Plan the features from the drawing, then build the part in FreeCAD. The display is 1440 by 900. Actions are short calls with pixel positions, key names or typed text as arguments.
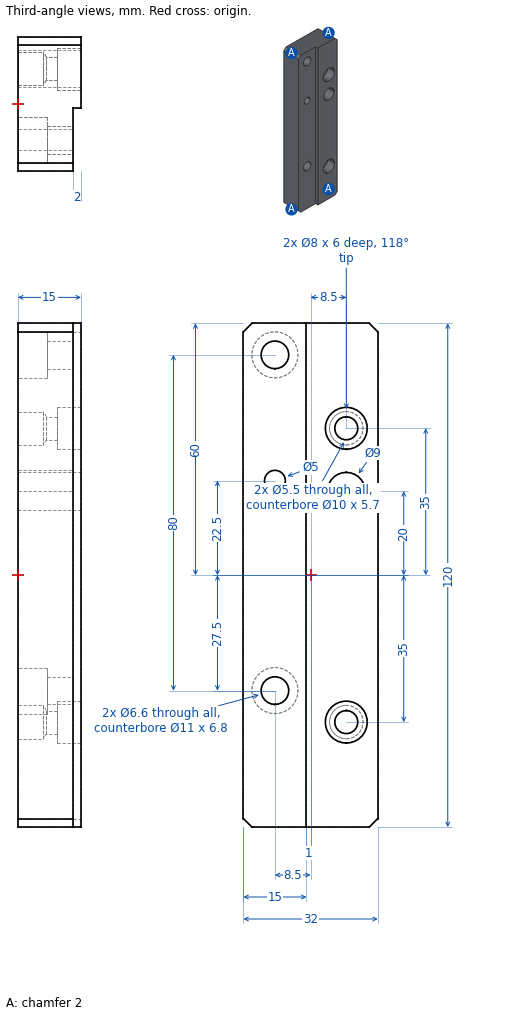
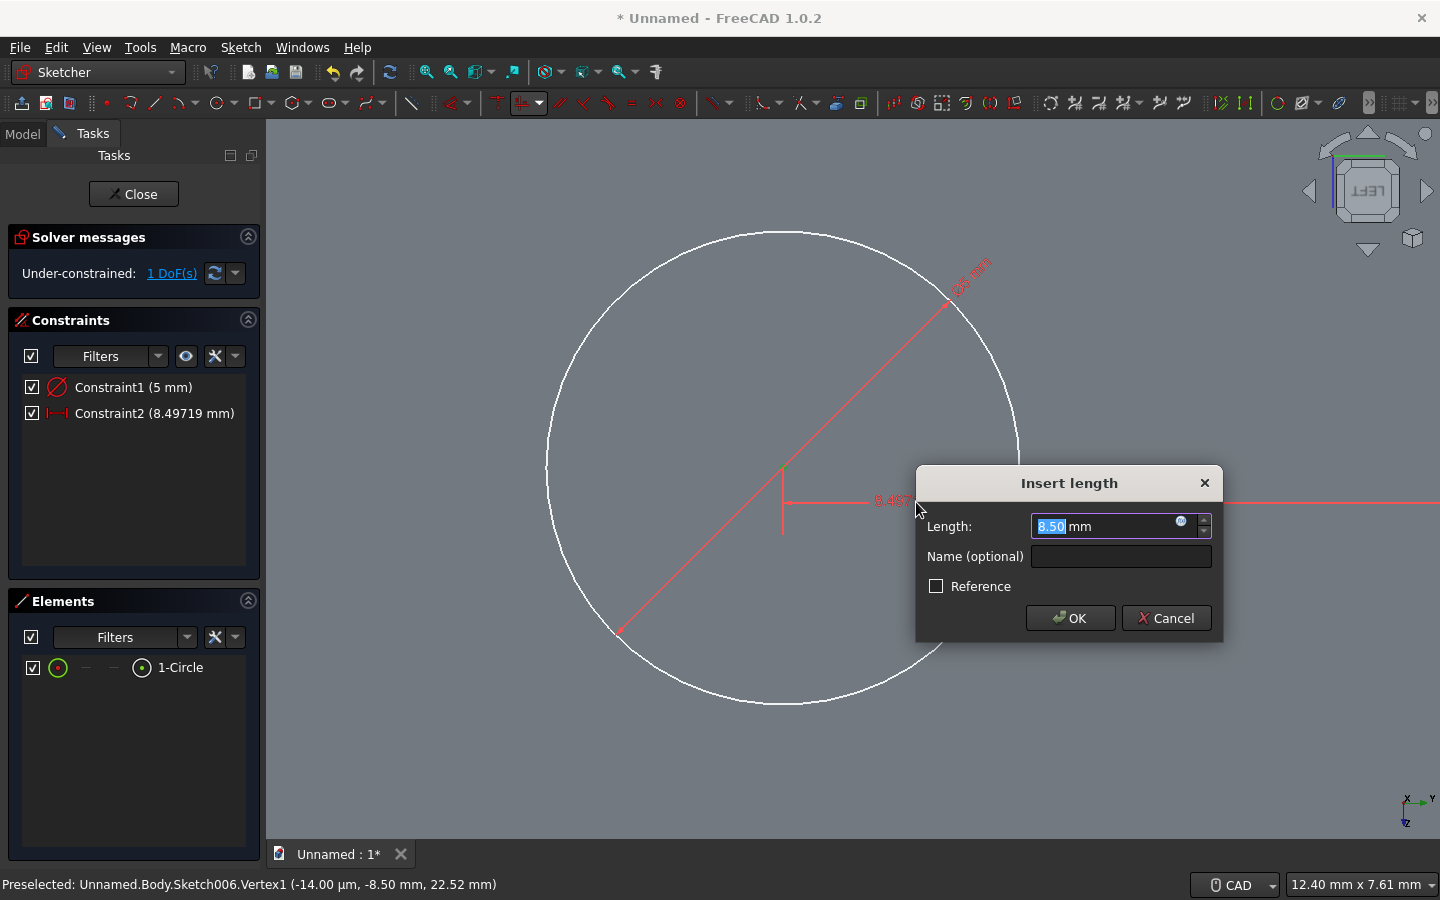
text(8.5)
key(Return)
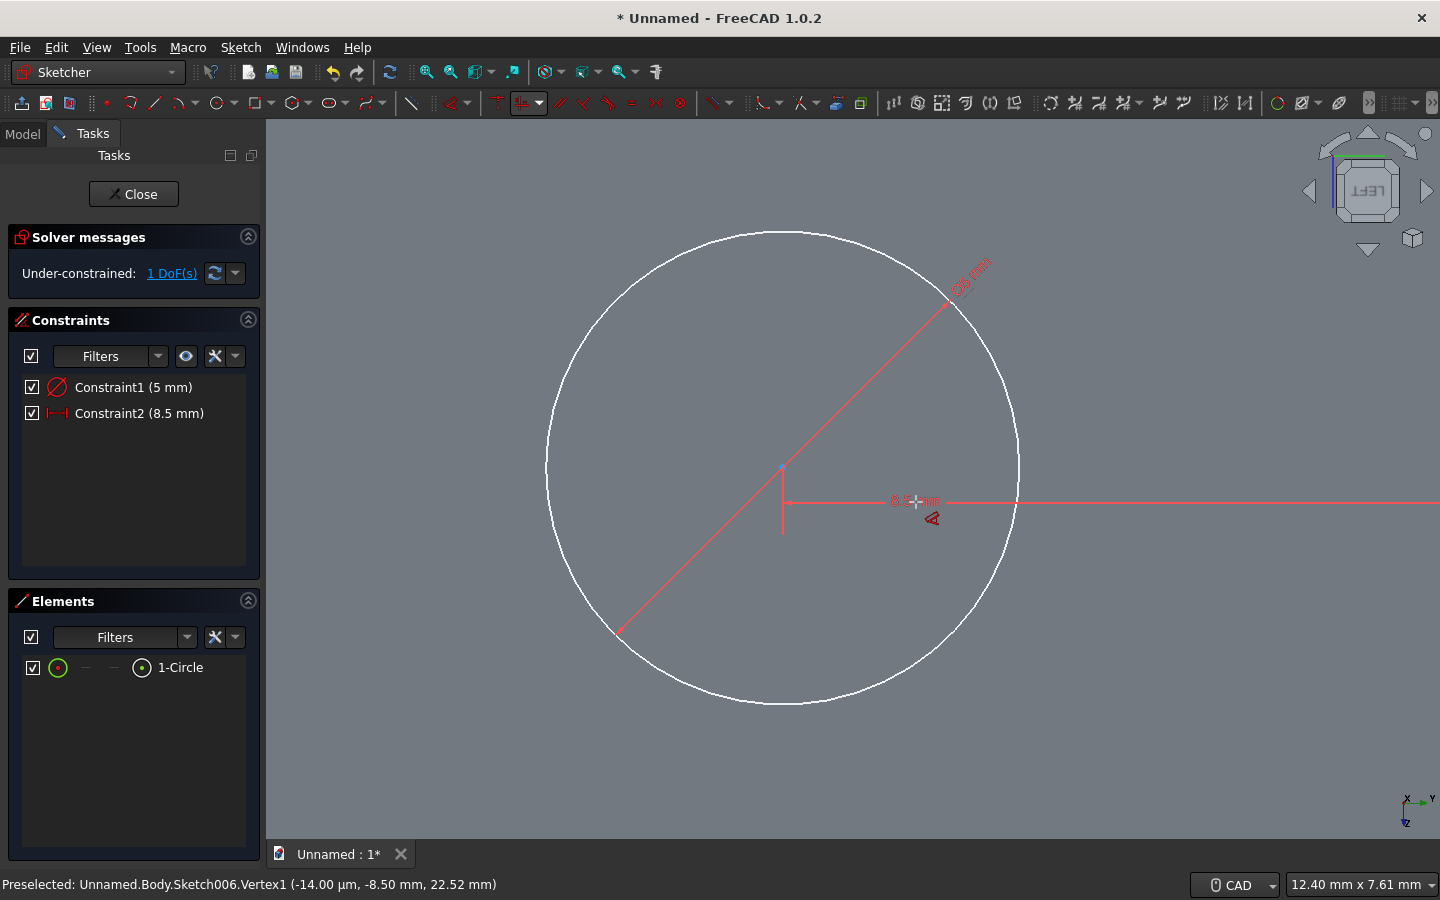
click(783, 468)
click(749, 307)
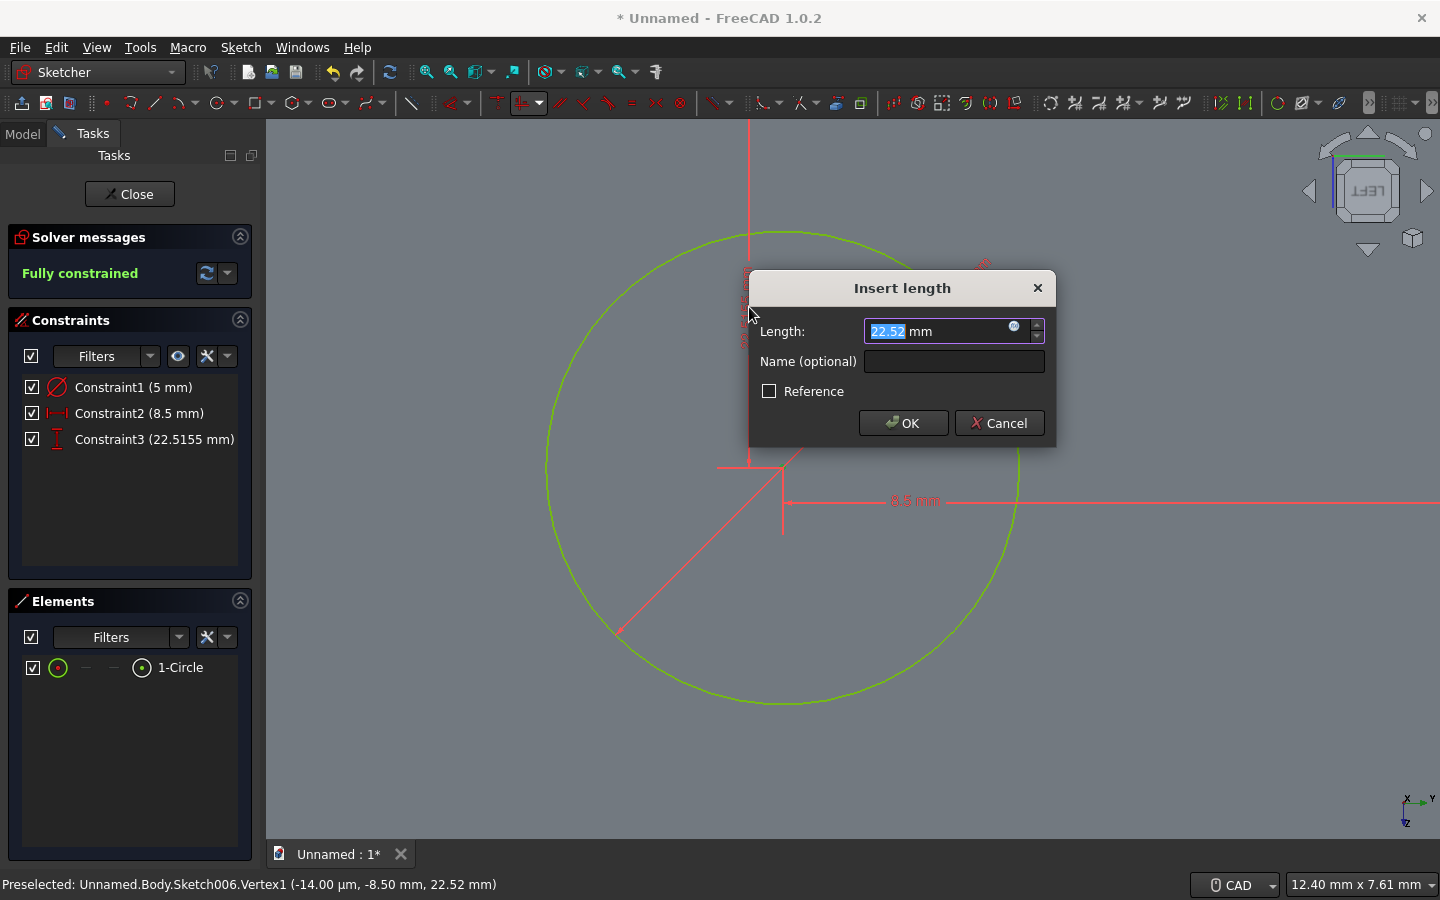
text(22.5)
key(Return)
key(Escape)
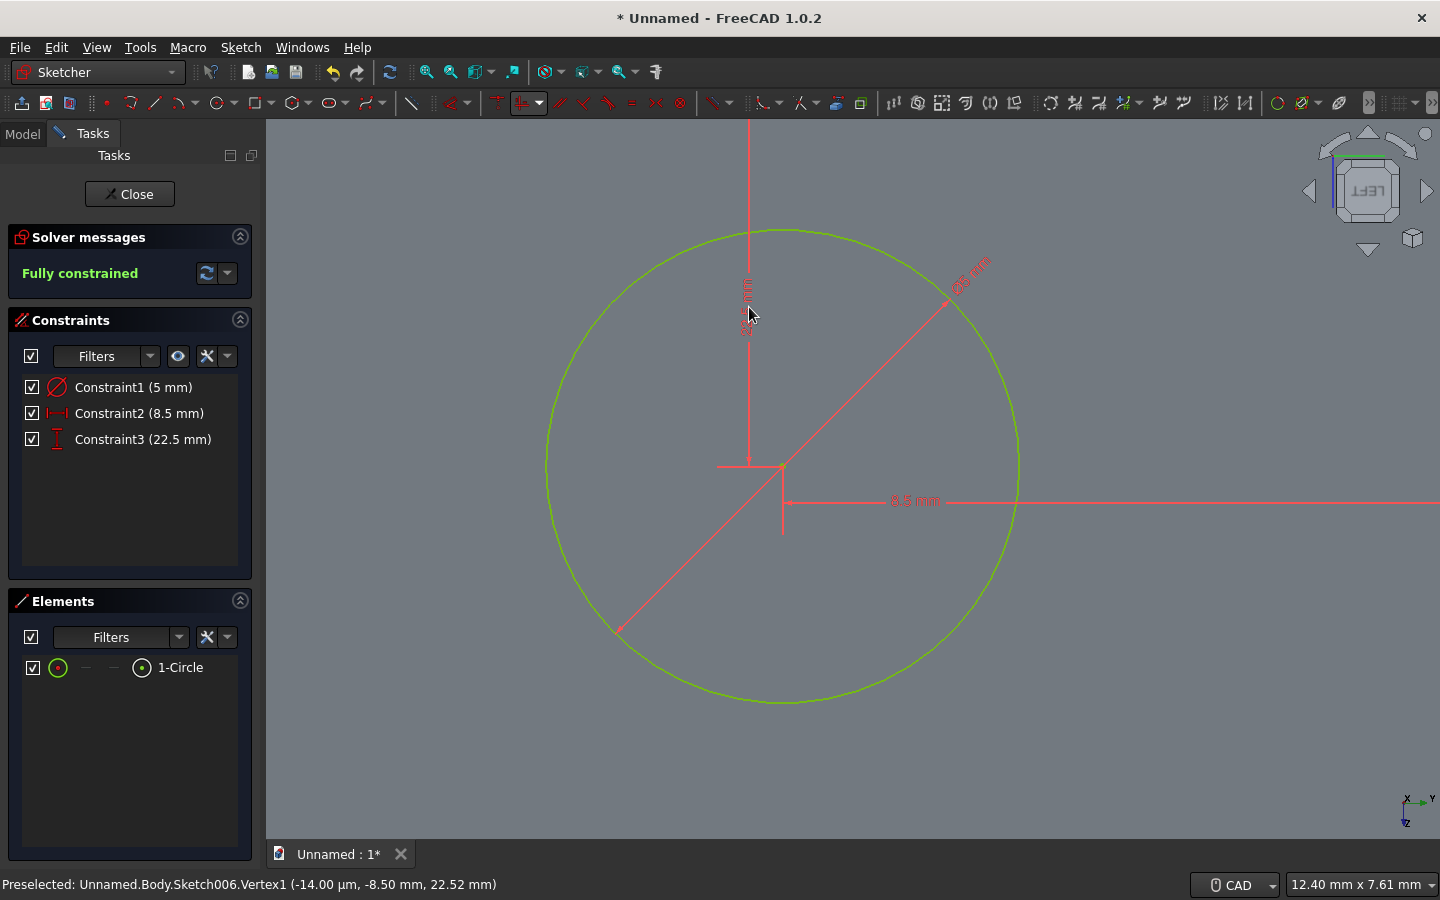
click(130, 194)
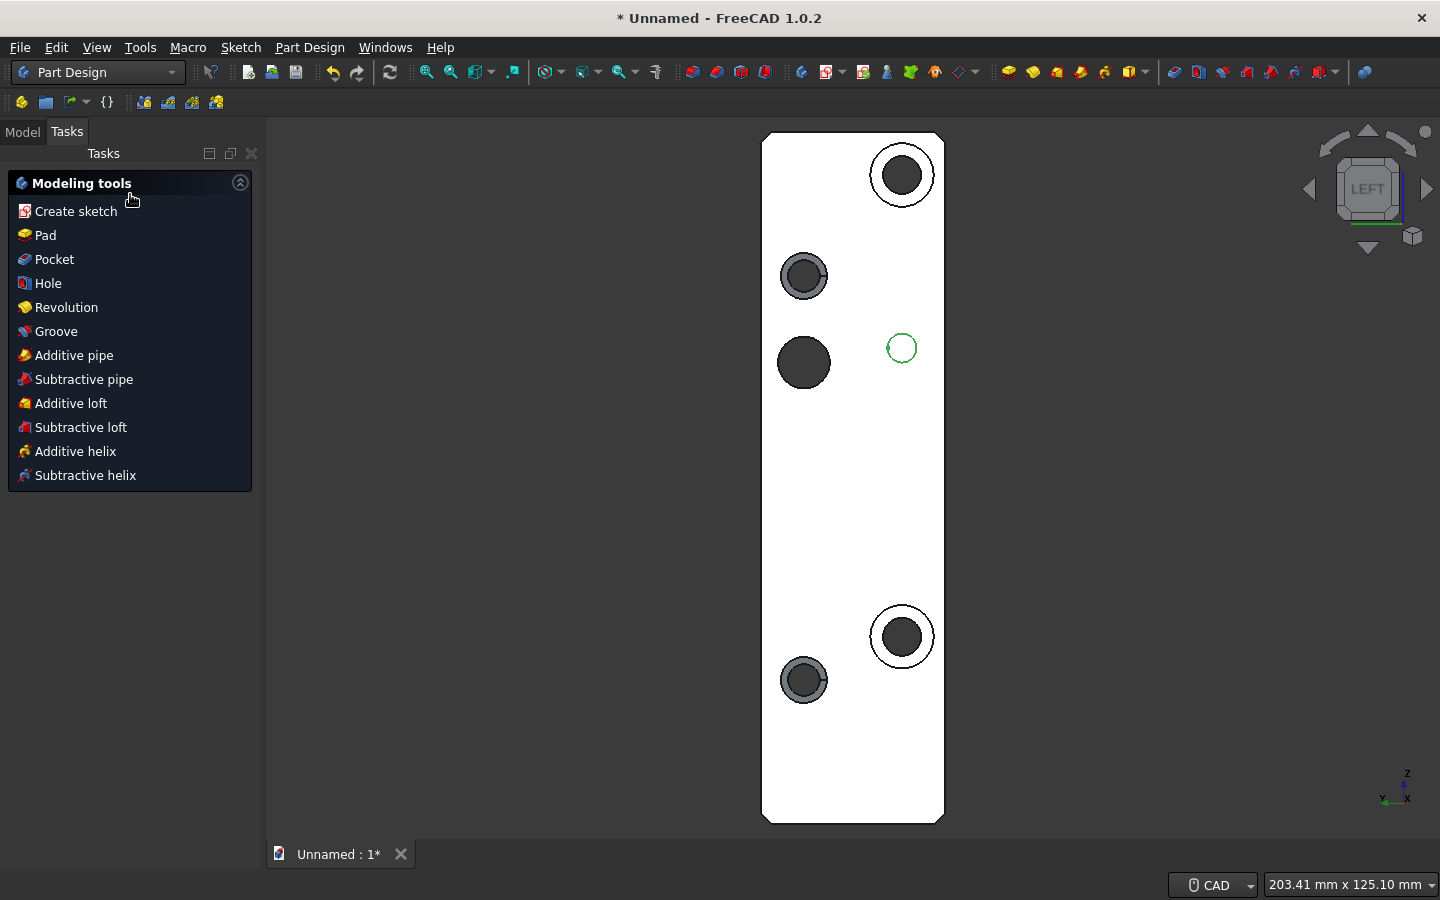
click(1176, 72)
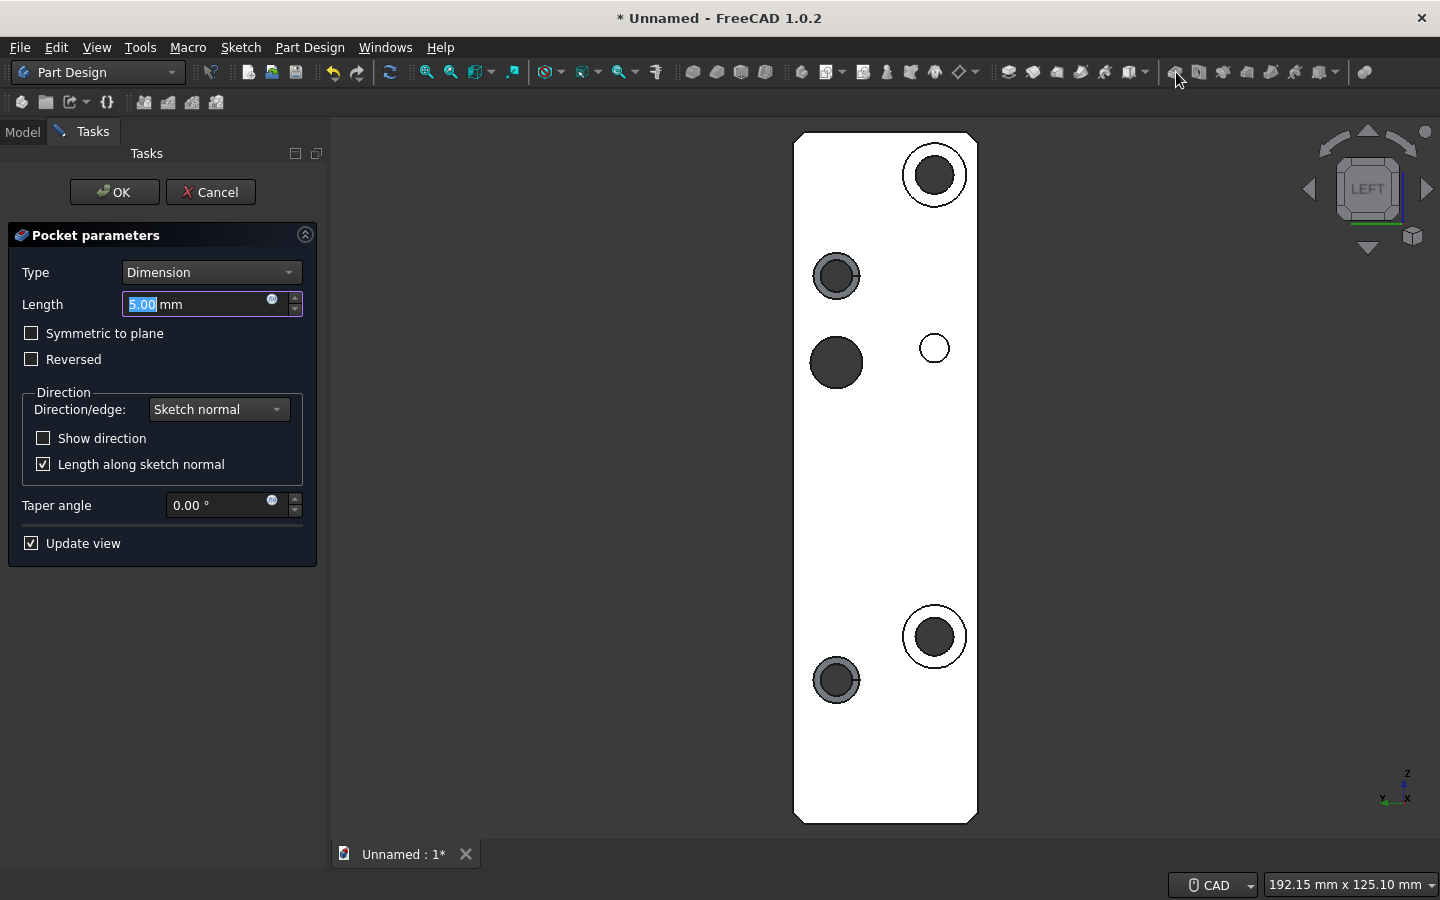
click(212, 272)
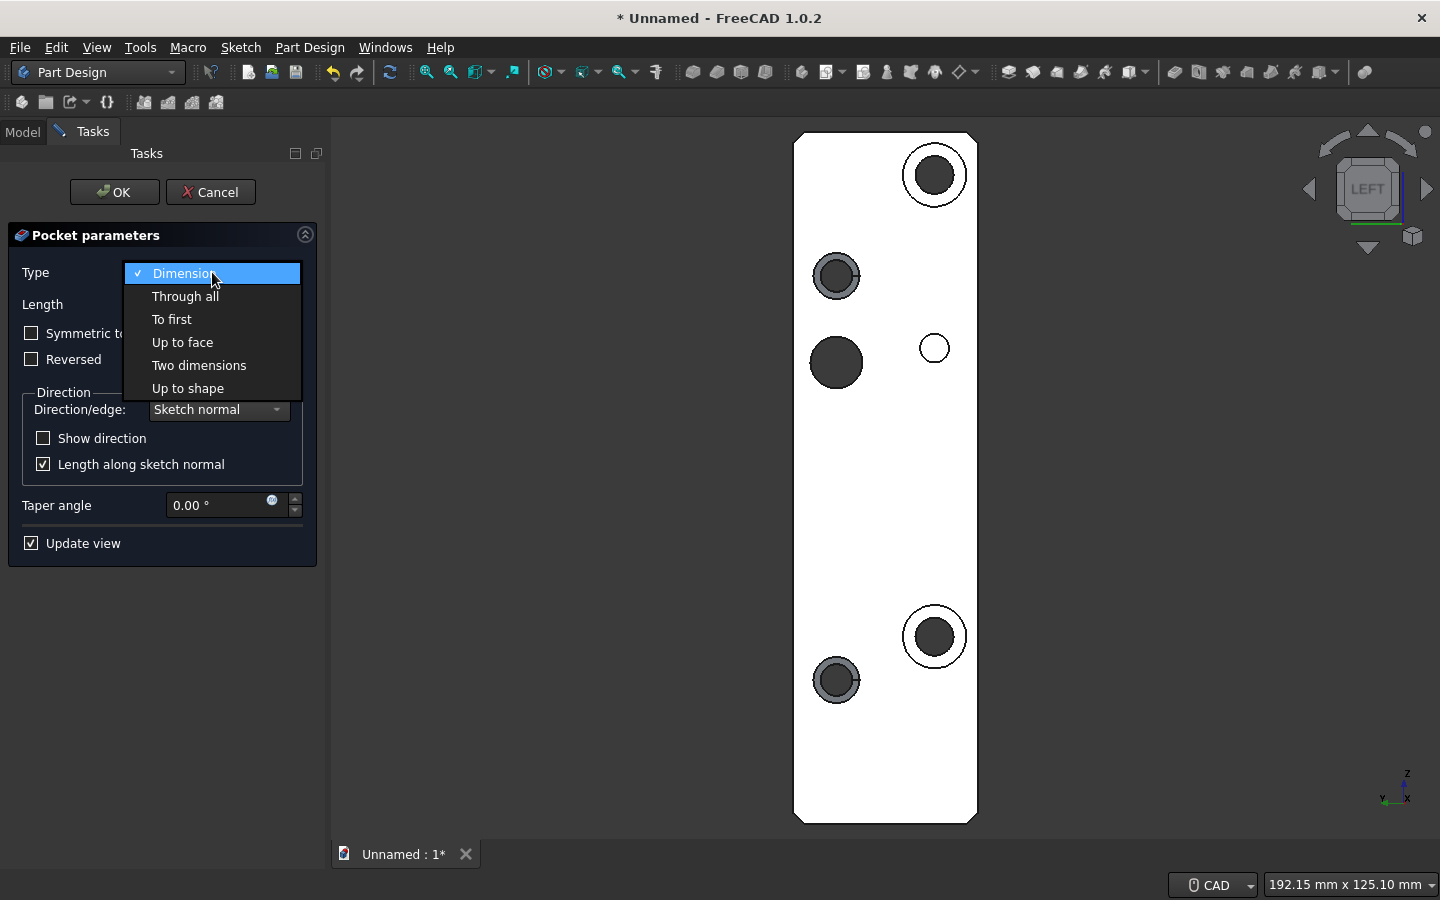
click(212, 296)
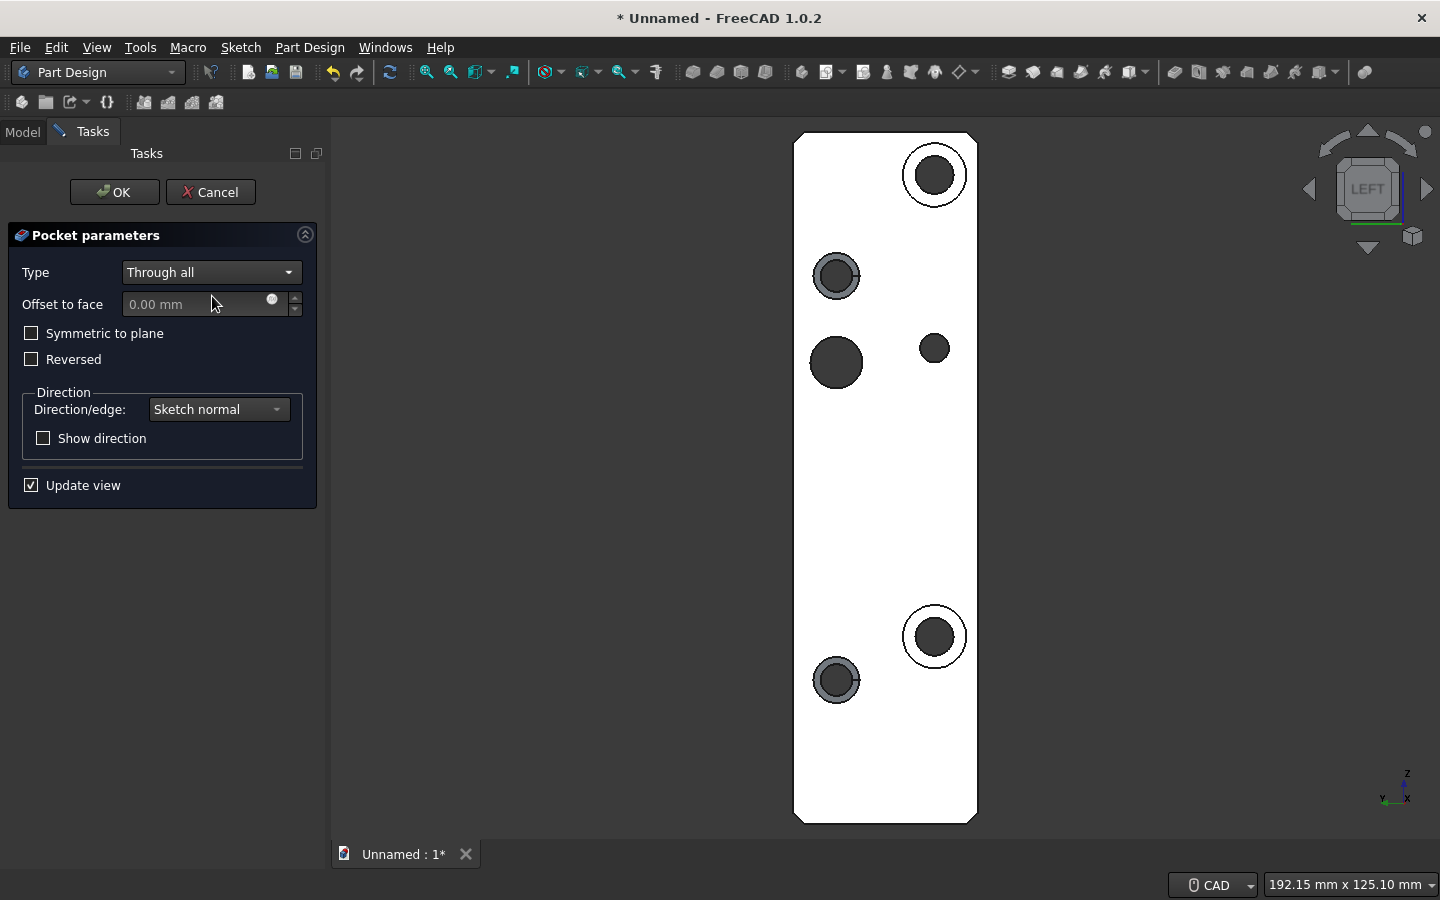
click(115, 192)